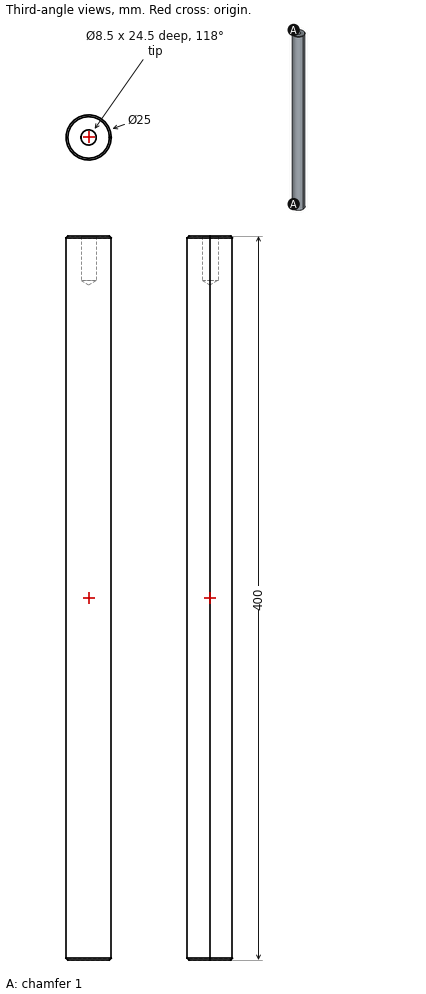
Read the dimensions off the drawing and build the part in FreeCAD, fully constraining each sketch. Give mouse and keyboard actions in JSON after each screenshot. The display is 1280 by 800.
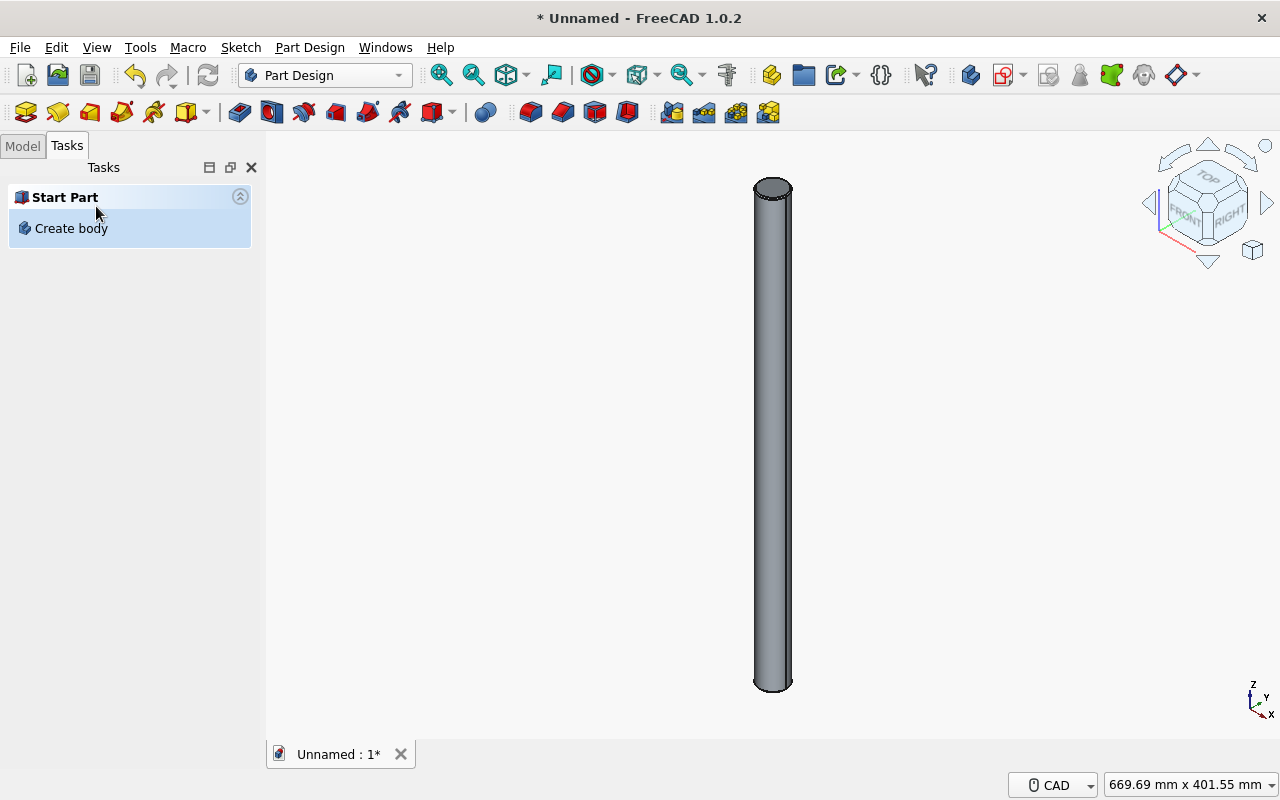
{"action": "left_click", "coordinate": [773, 187]}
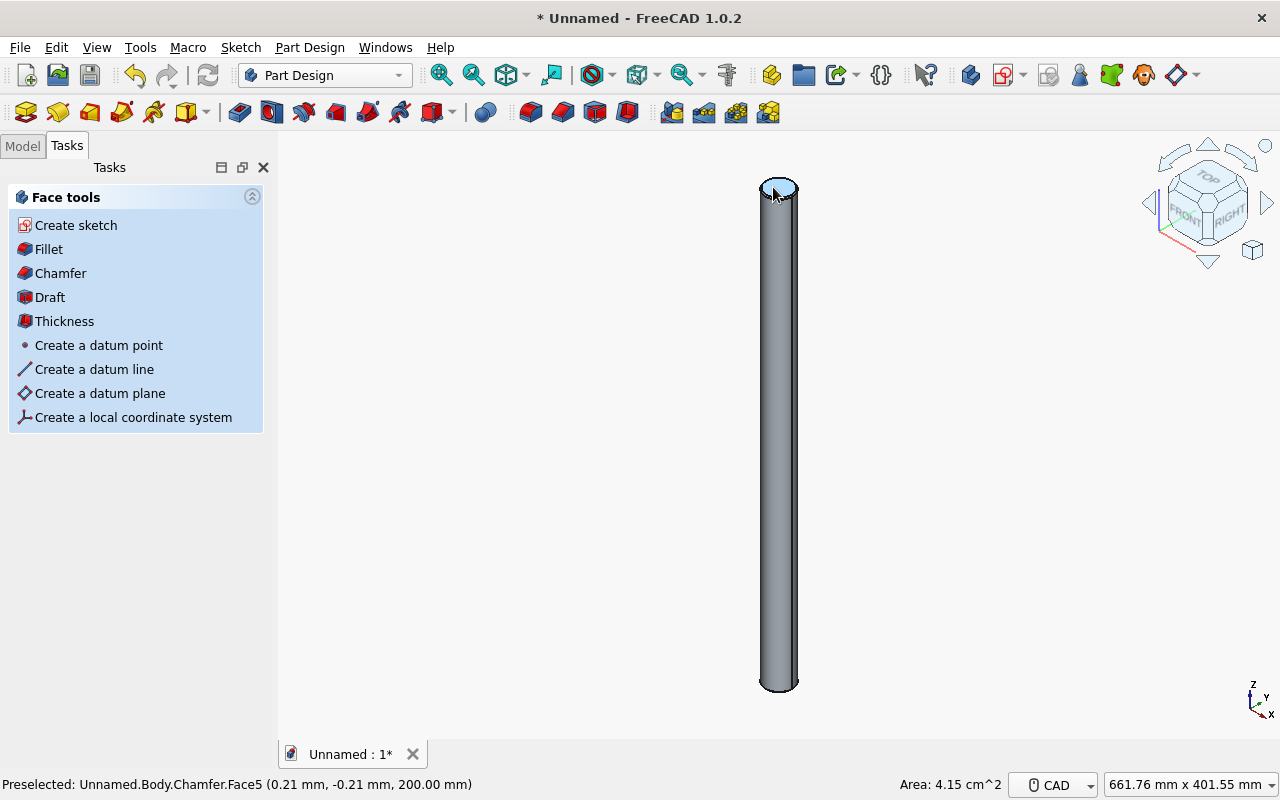
{"action": "left_click", "coordinate": [1004, 76]}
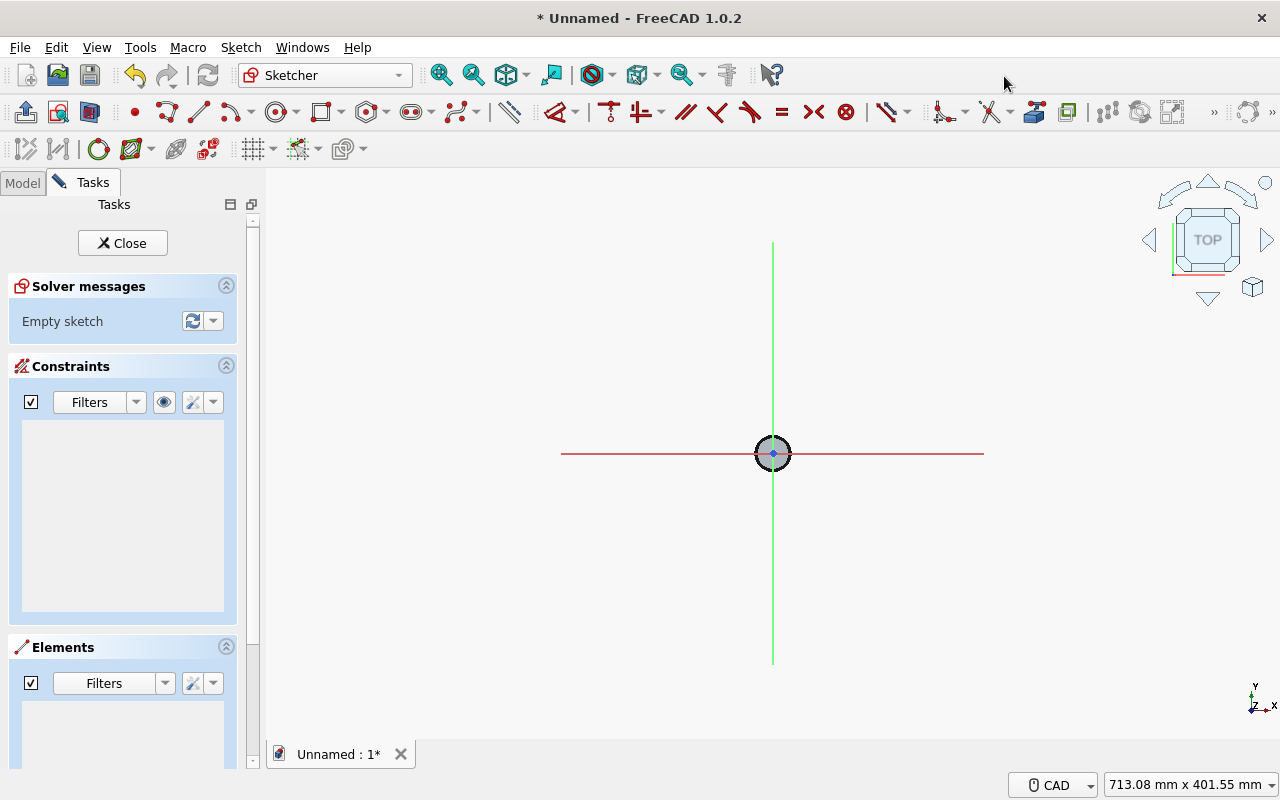
{"action": "scroll", "coordinate": [777, 454], "scroll_direction": "up", "scroll_amount": 15}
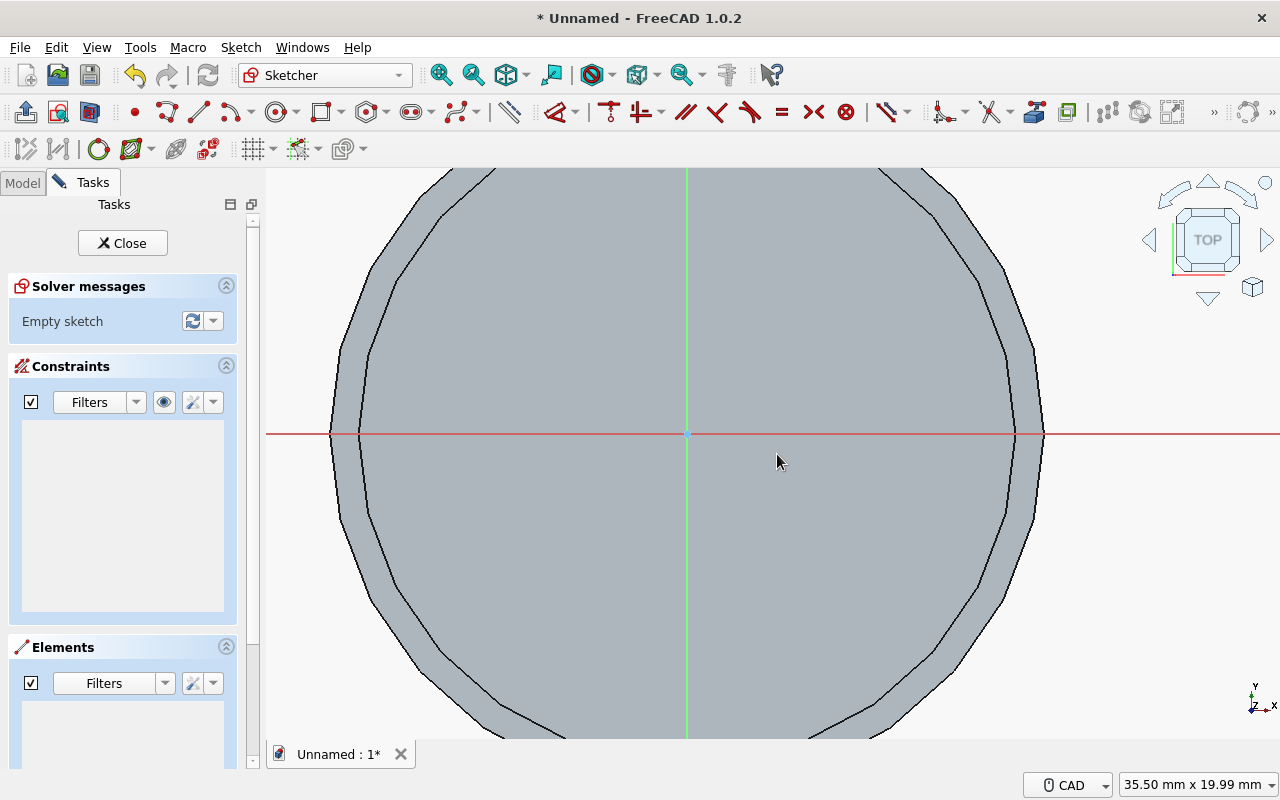
{"action": "scroll", "coordinate": [652, 396], "scroll_direction": "up", "scroll_amount": 2}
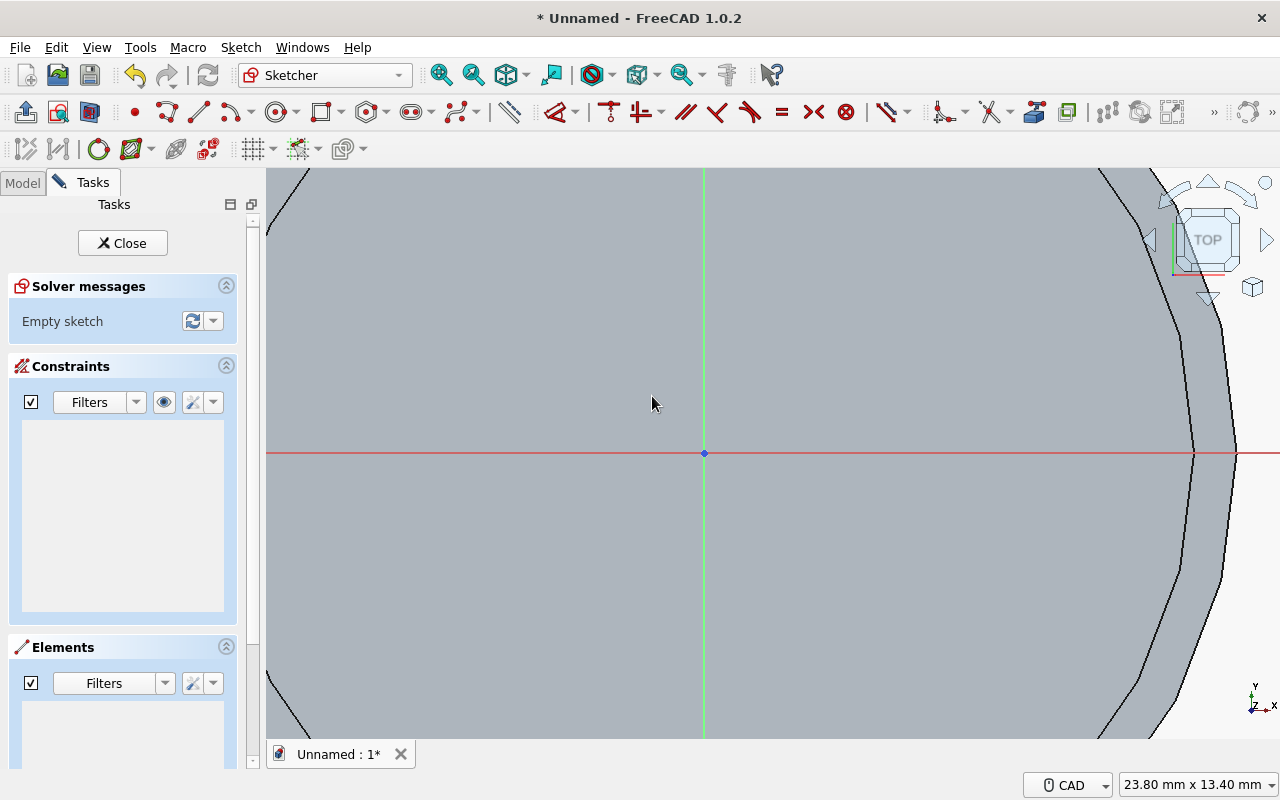
{"action": "left_click", "coordinate": [276, 112]}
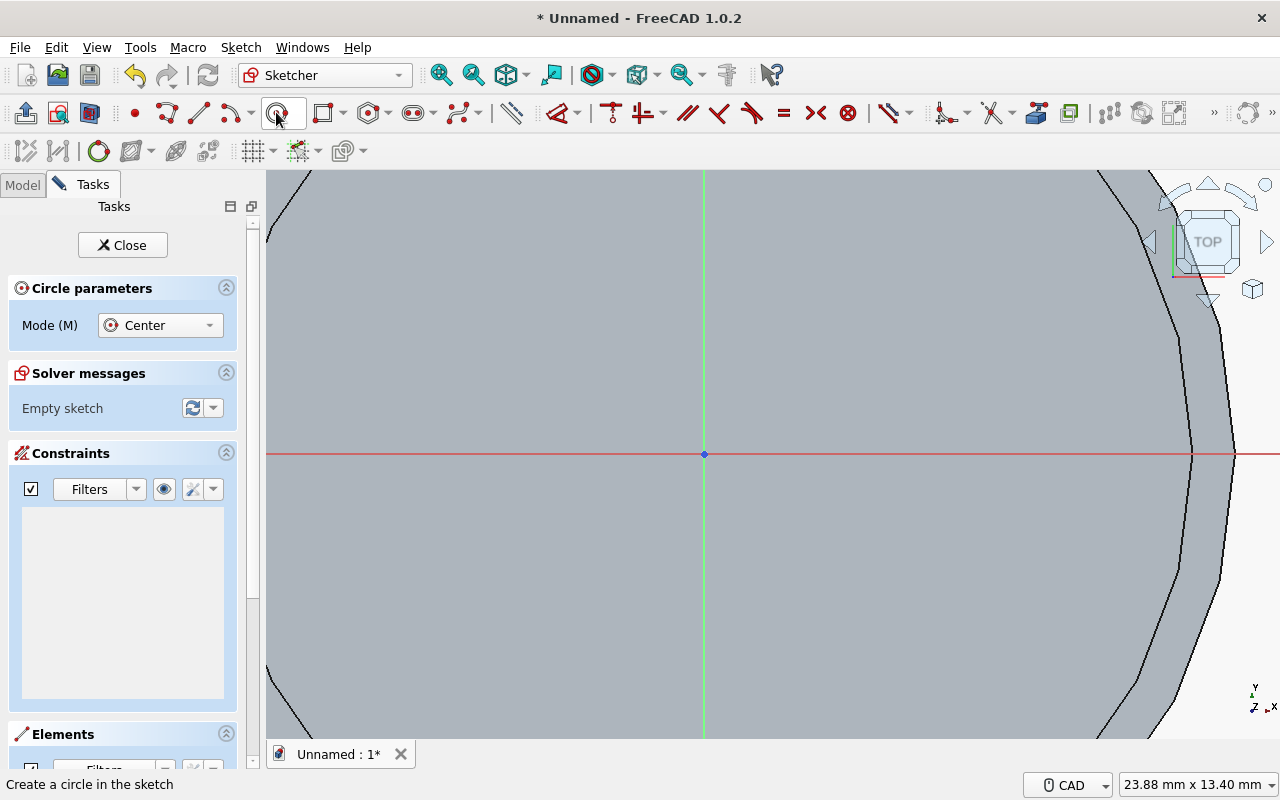
{"action": "left_click", "coordinate": [704, 454]}
{"action": "mouse_move", "coordinate": [832, 326]}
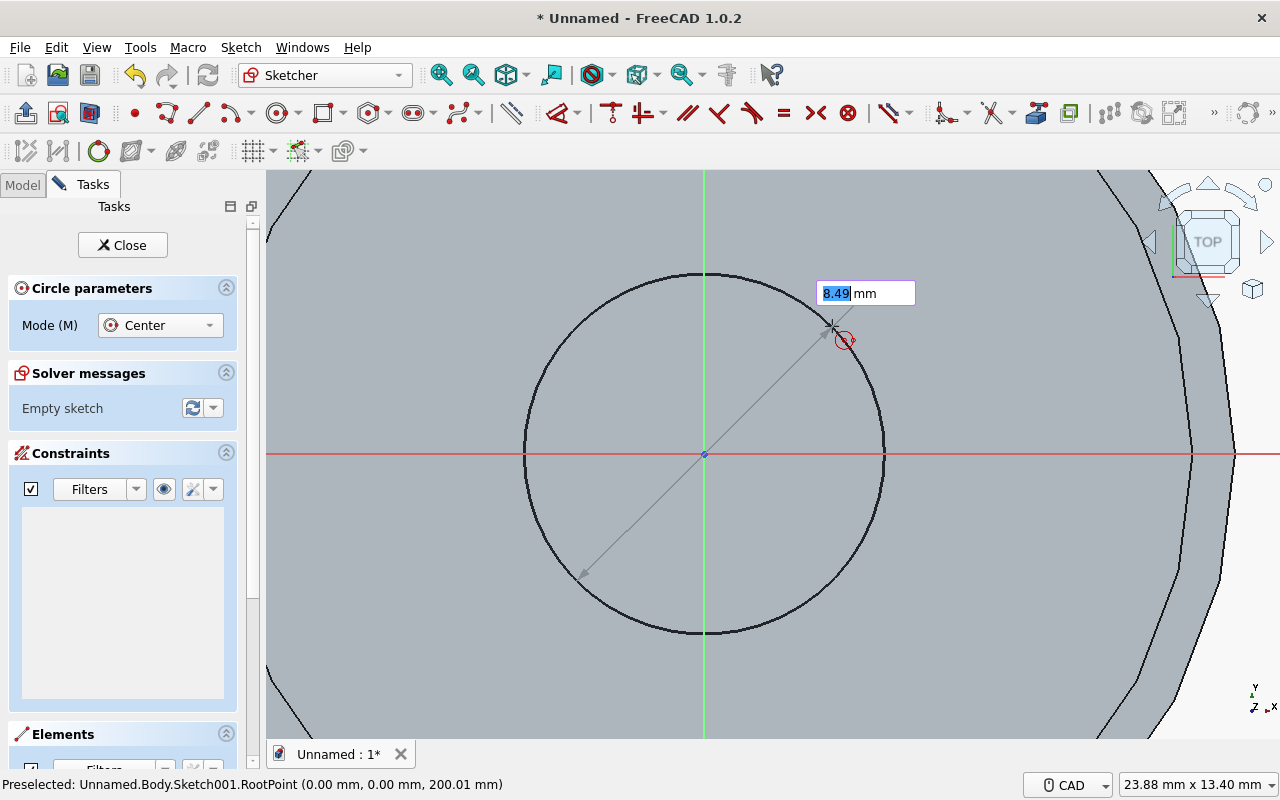
{"action": "type", "text": "8.5"}
{"action": "key", "text": "Return"}
{"action": "key", "text": "Escape"}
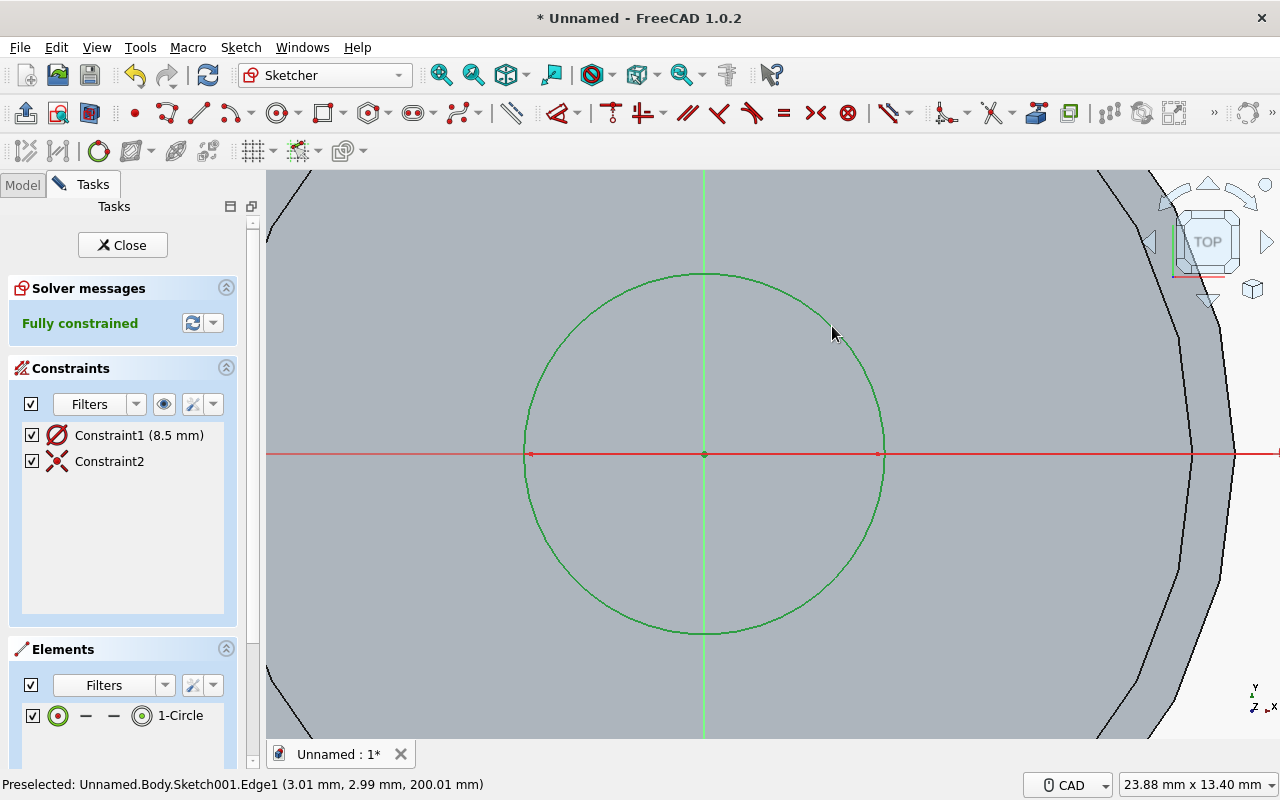
{"action": "left_click", "coordinate": [123, 245]}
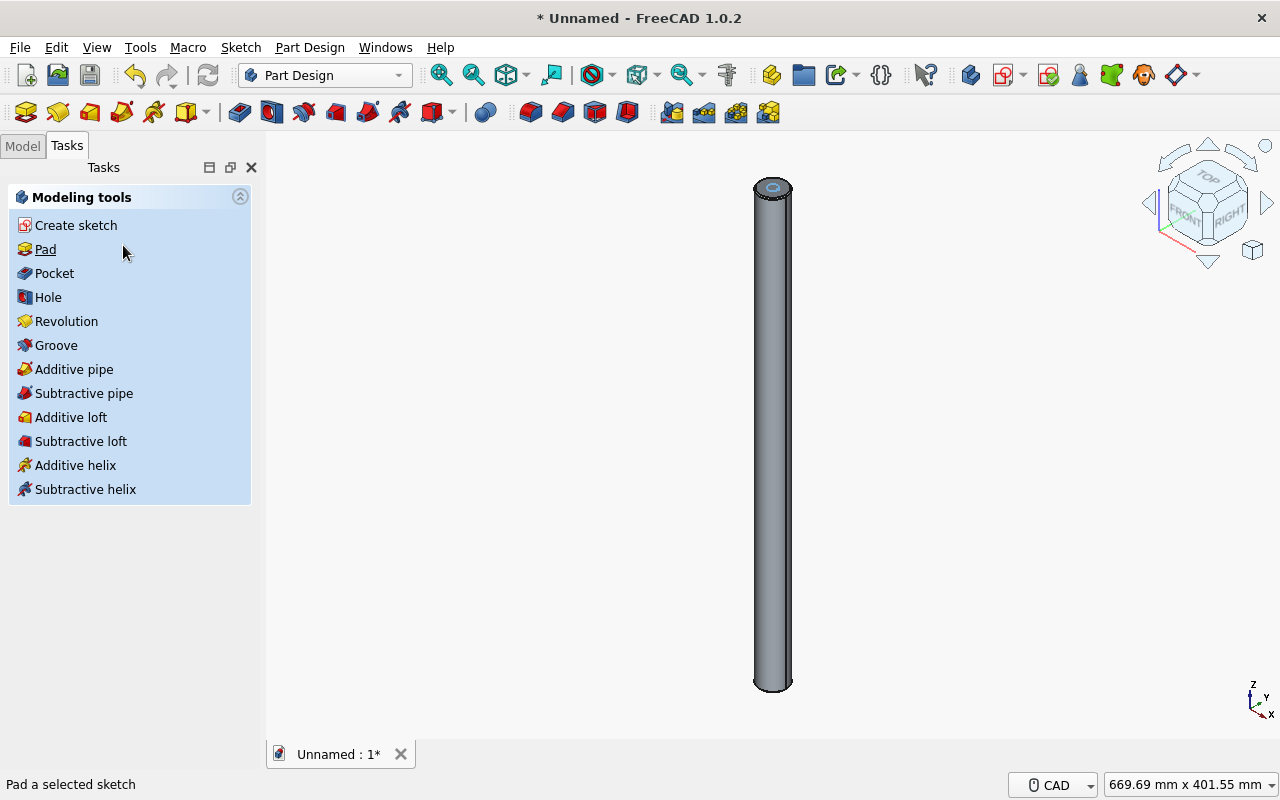
{"action": "left_click", "coordinate": [272, 112]}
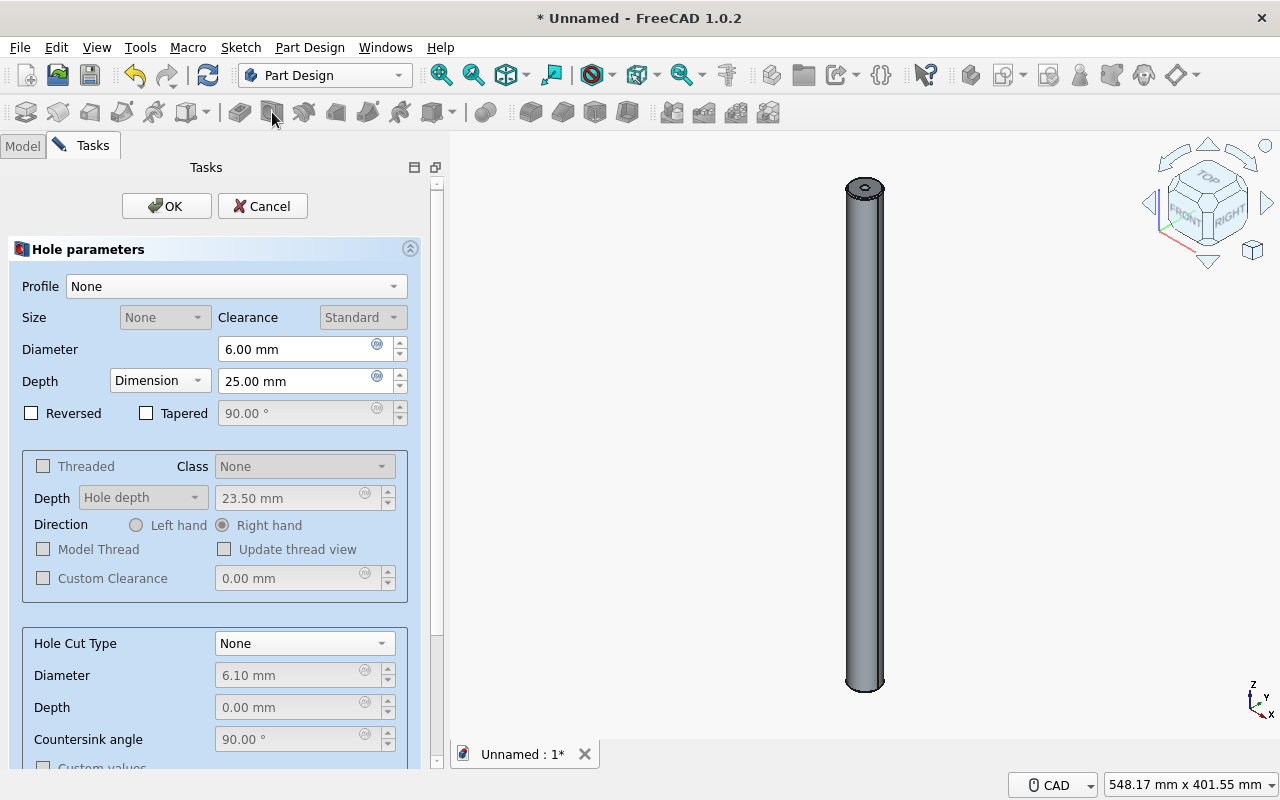
{"action": "triple_click", "coordinate": [305, 349]}